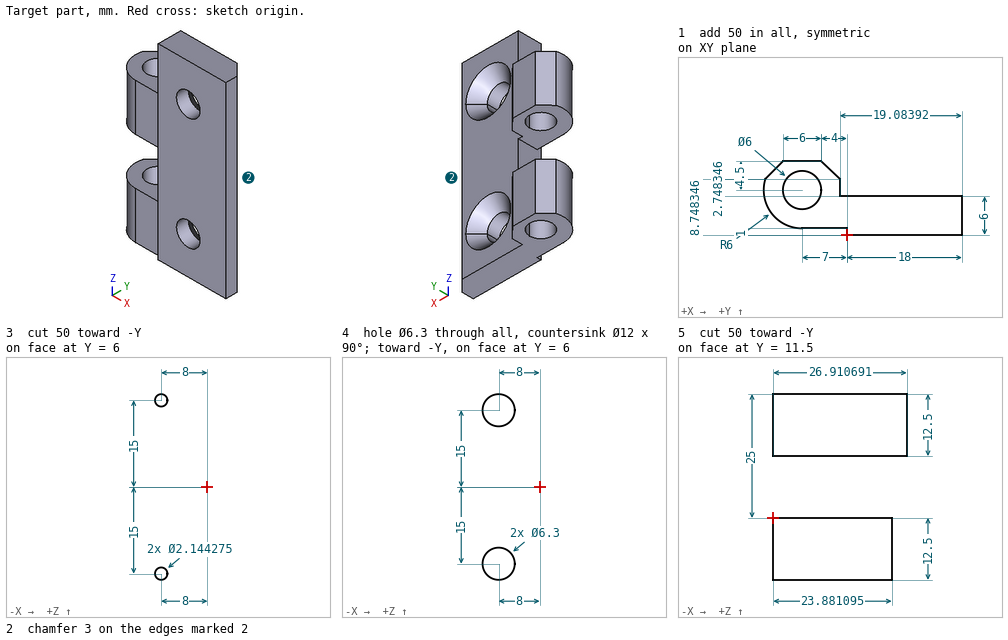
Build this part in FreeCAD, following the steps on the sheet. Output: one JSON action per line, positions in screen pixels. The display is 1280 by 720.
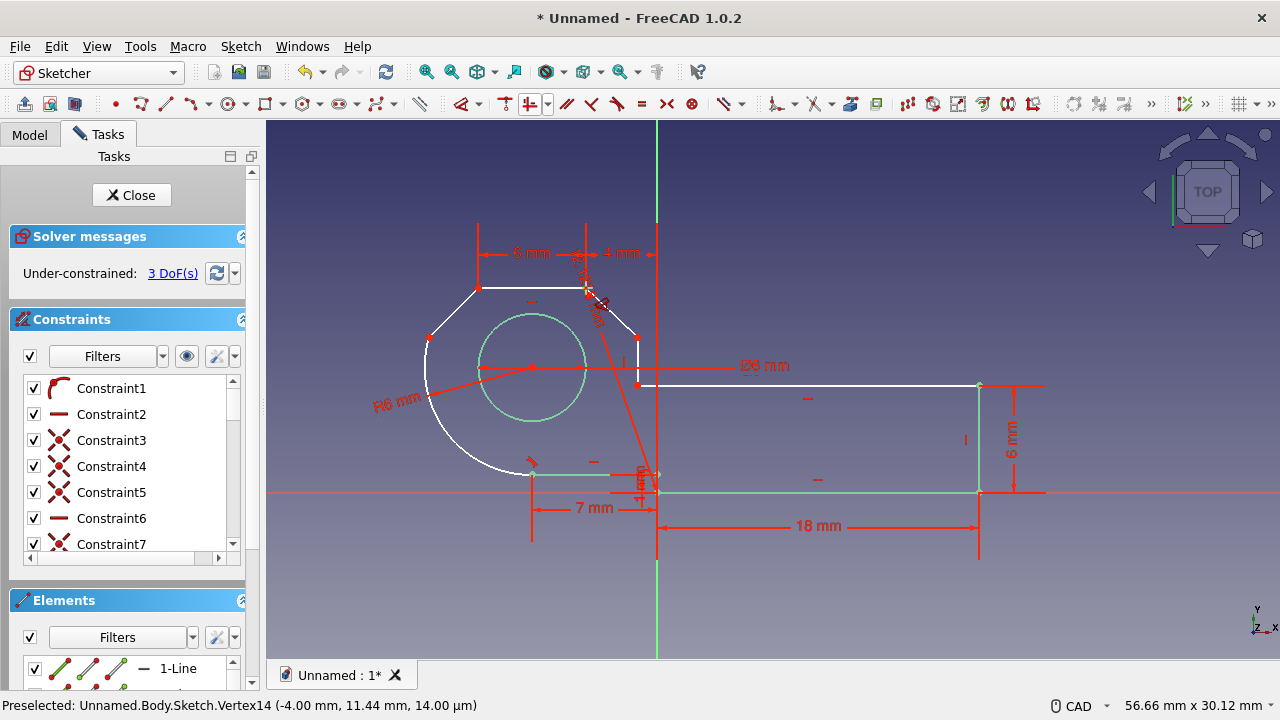
{"action": "left_click", "coordinate": [532, 368]}
{"action": "left_click", "coordinate": [498, 310]}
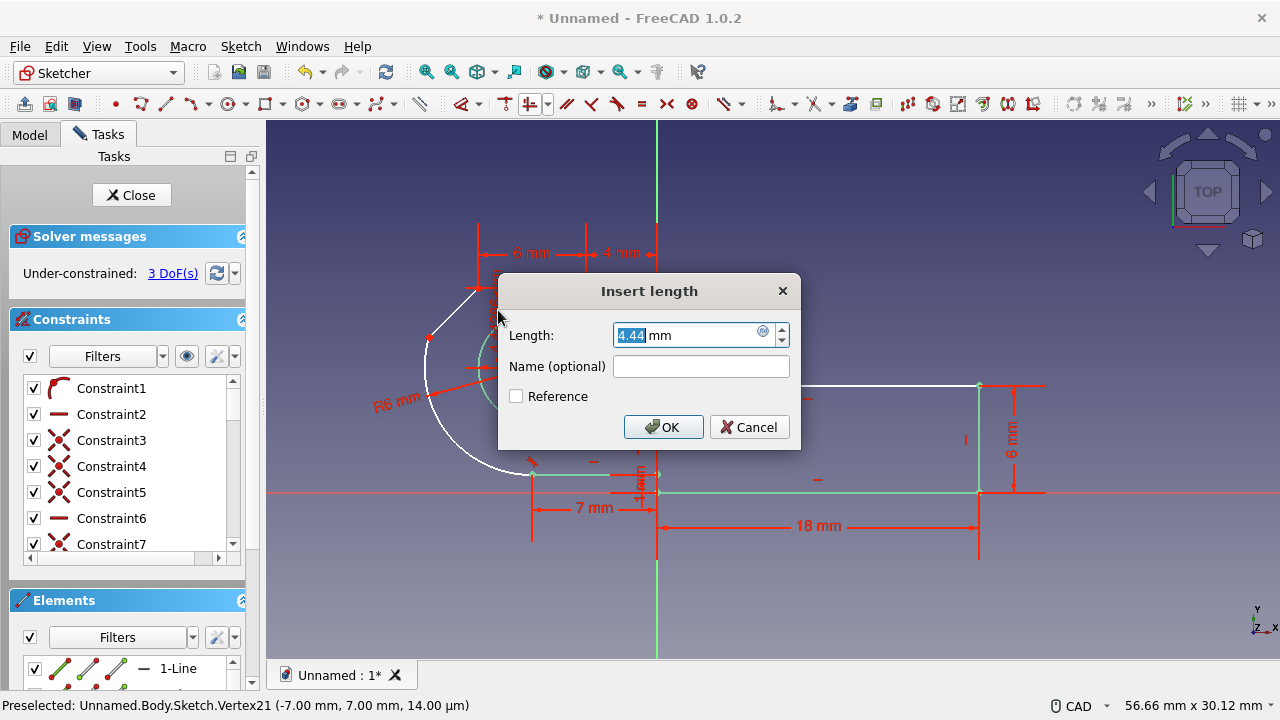
{"action": "type", "text": "4.5"}
{"action": "key", "text": "Return"}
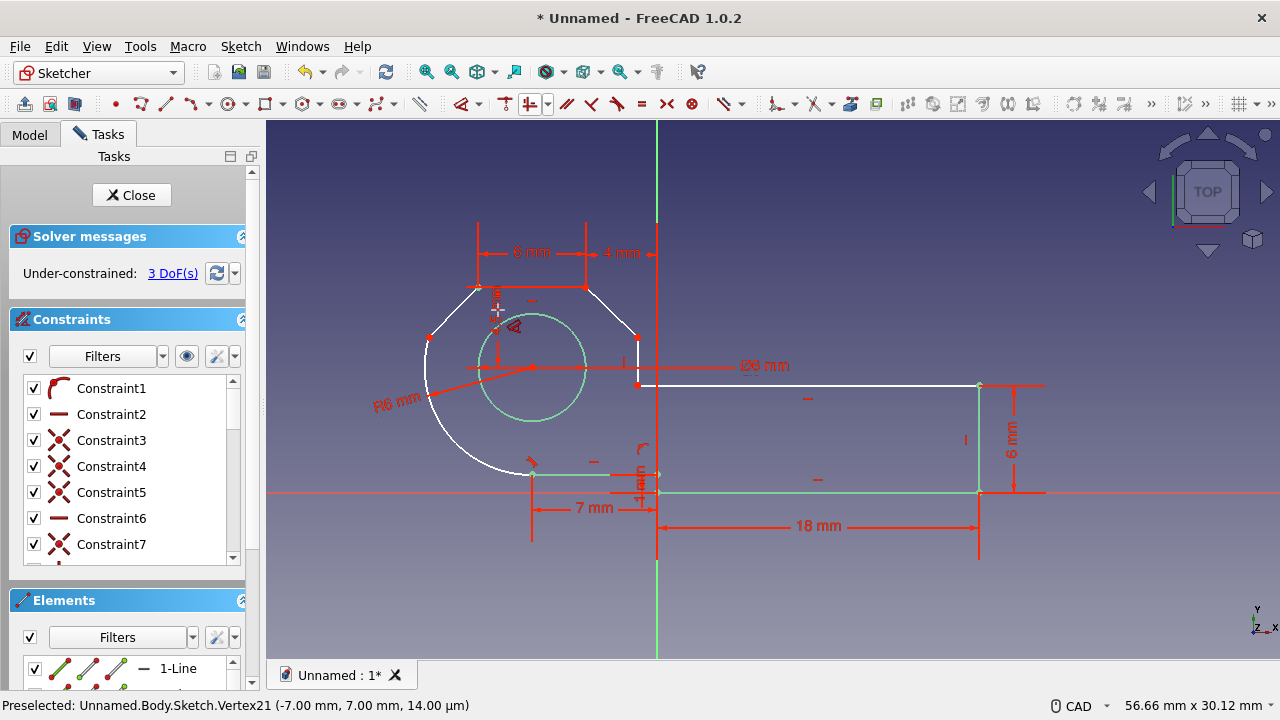
{"action": "left_click", "coordinate": [877, 386]}
{"action": "left_click", "coordinate": [809, 352]}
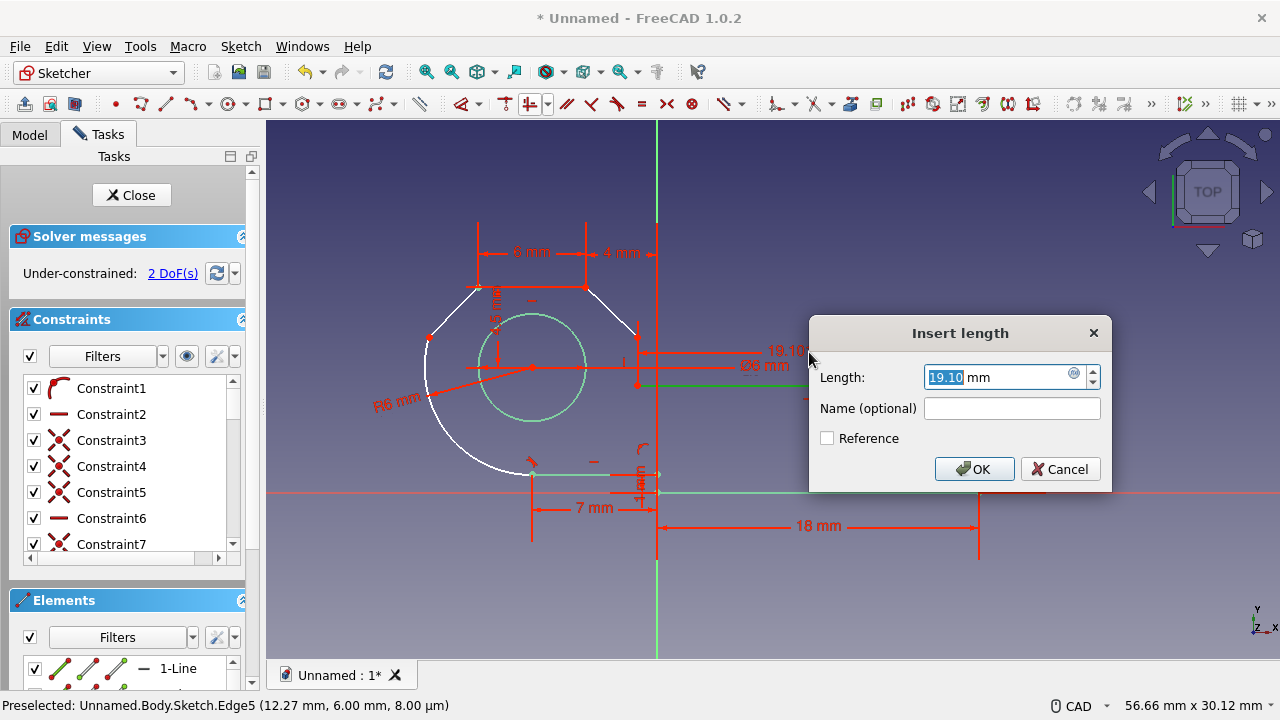
{"action": "type", "text": "19.08392"}
{"action": "key", "text": "Return"}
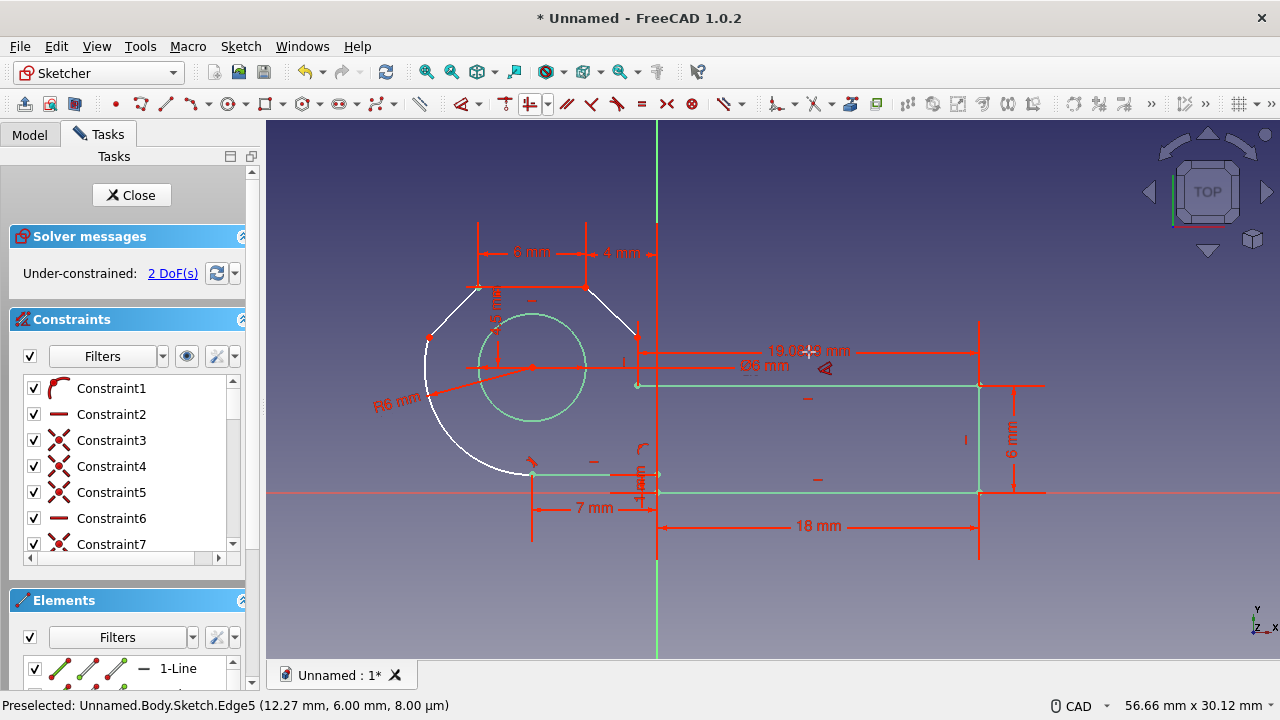
{"action": "left_click", "coordinate": [638, 371]}
{"action": "left_click", "coordinate": [604, 361]}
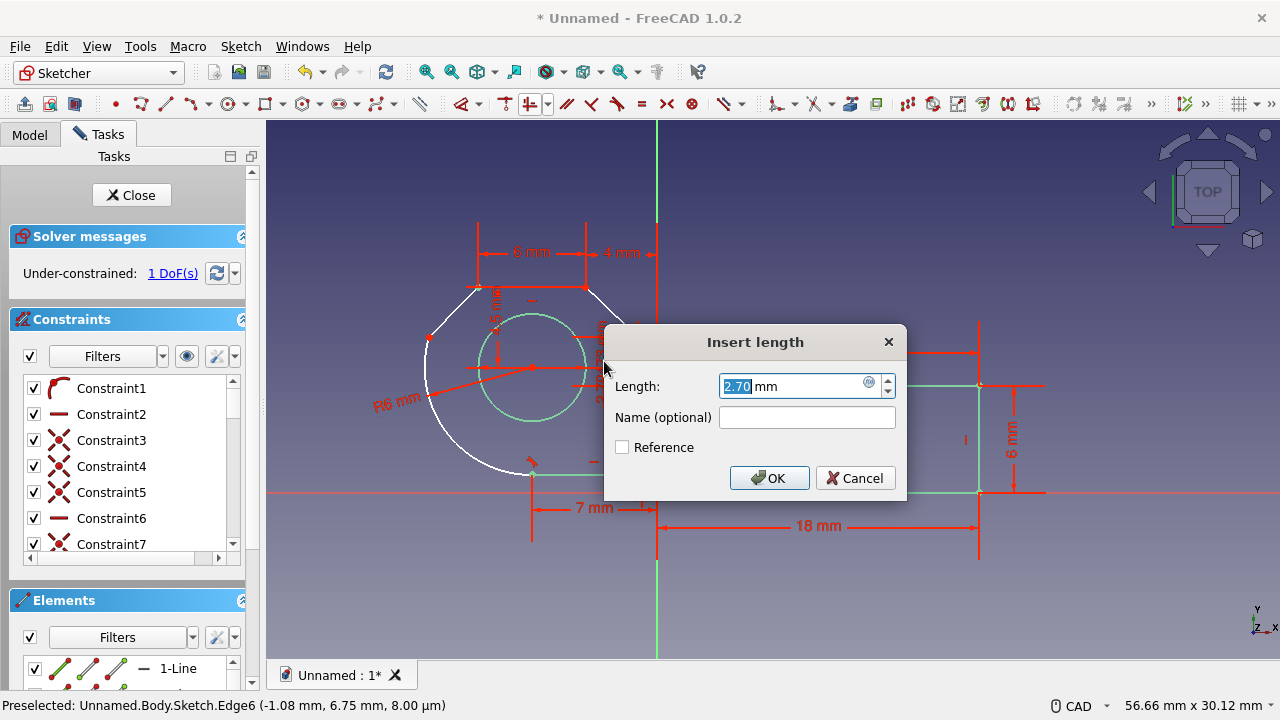
{"action": "type", "text": "2.748346"}
{"action": "key", "text": "Return"}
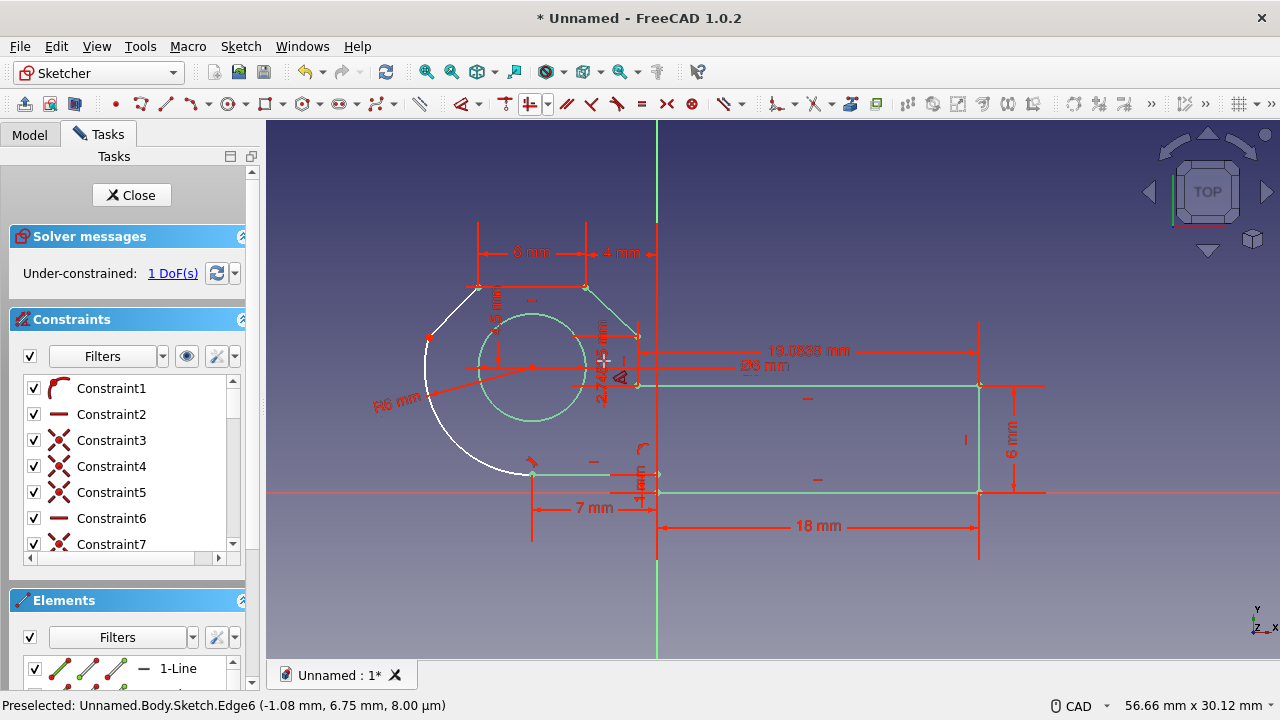
{"action": "left_click", "coordinate": [429, 337]}
{"action": "left_click", "coordinate": [395, 379]}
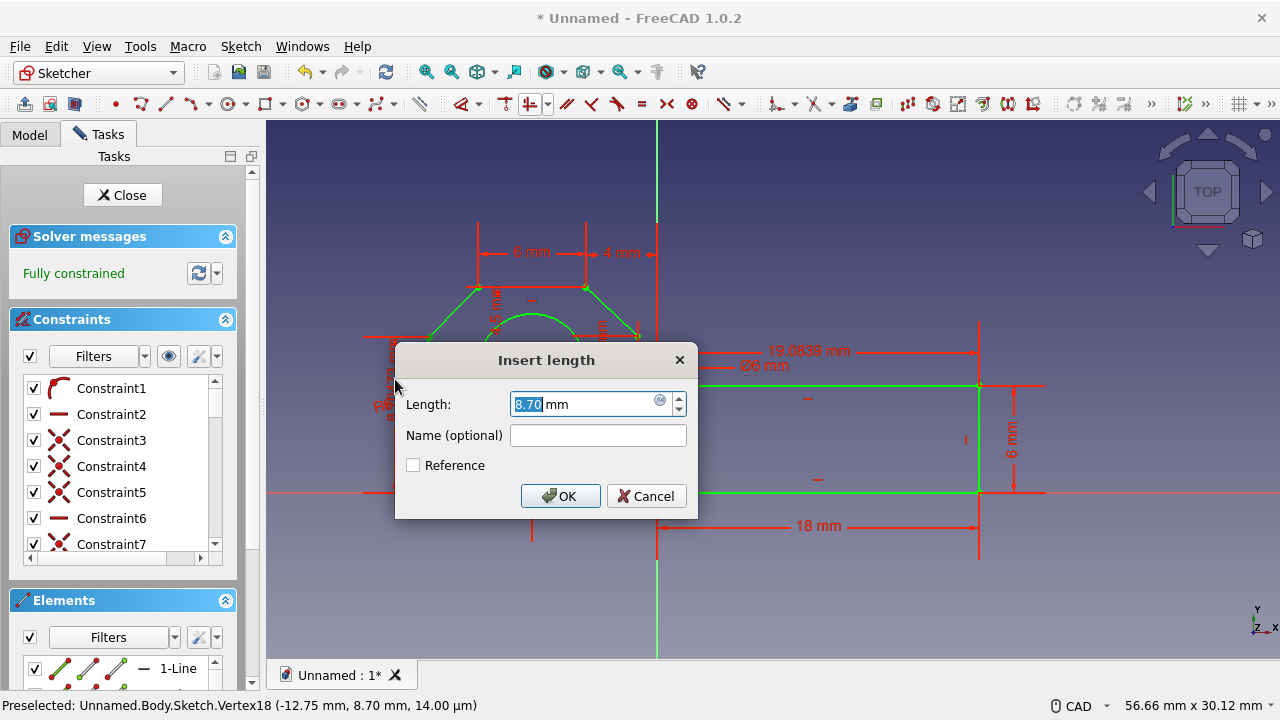
{"action": "type", "text": "8.748346"}
{"action": "key", "text": "Return"}
{"action": "key", "text": "Escape"}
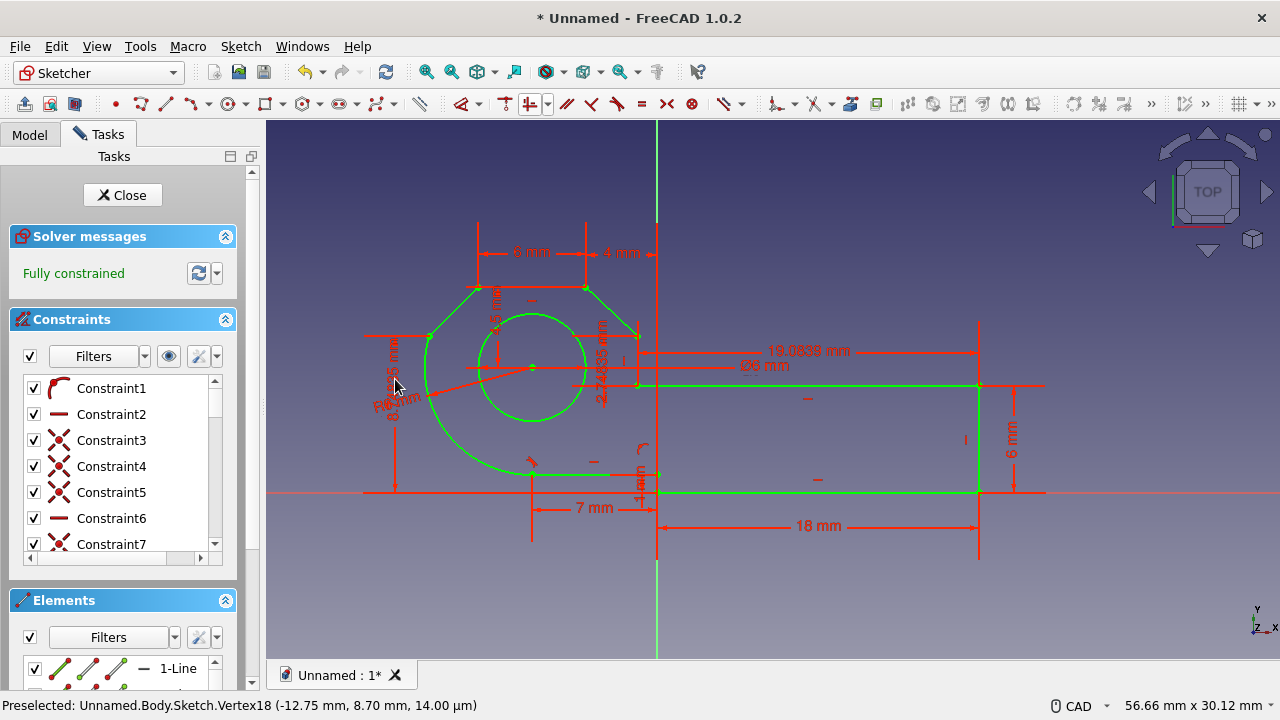
{"action": "left_click", "coordinate": [123, 195]}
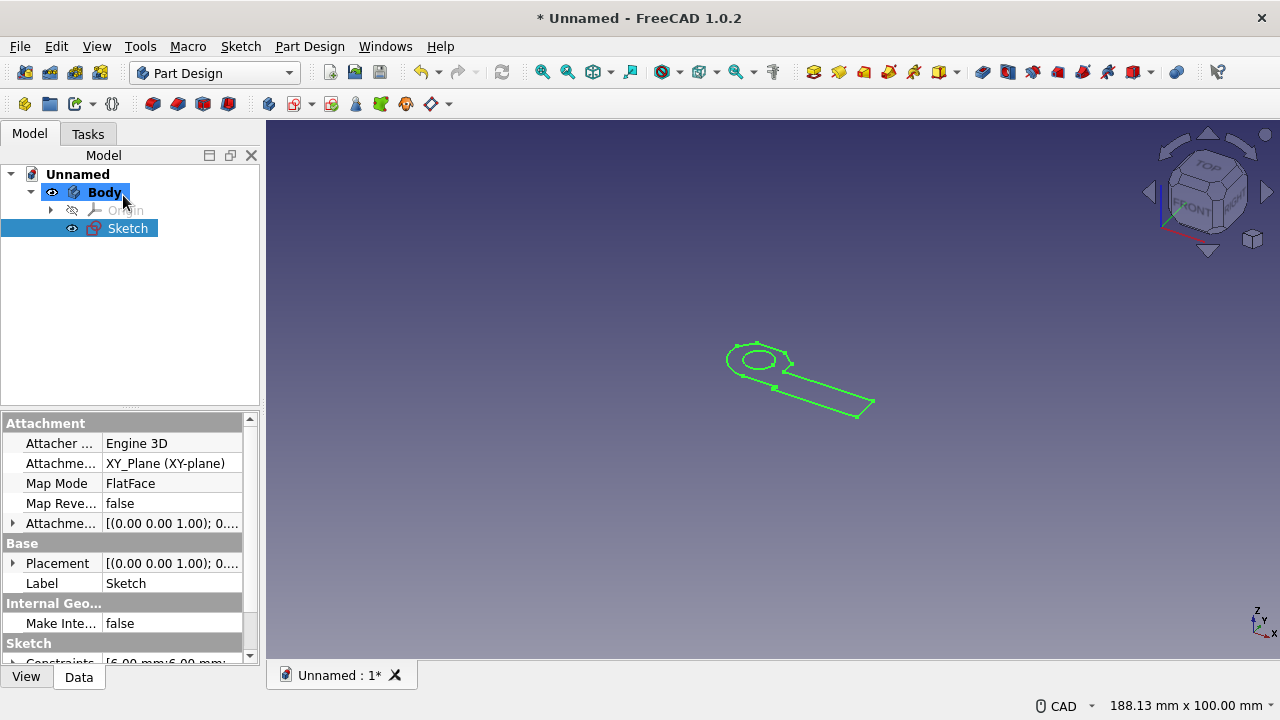
{"action": "left_click", "coordinate": [814, 72]}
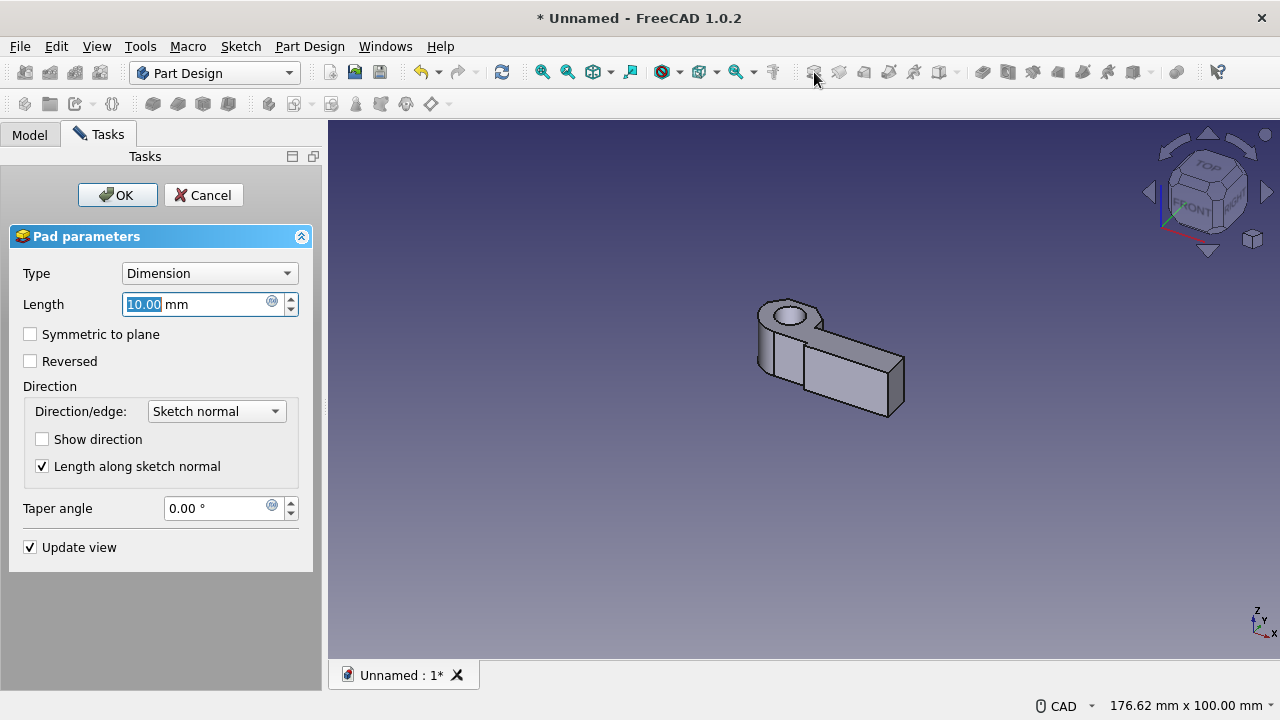
{"action": "type", "text": "50"}
{"action": "key", "text": "Tab"}